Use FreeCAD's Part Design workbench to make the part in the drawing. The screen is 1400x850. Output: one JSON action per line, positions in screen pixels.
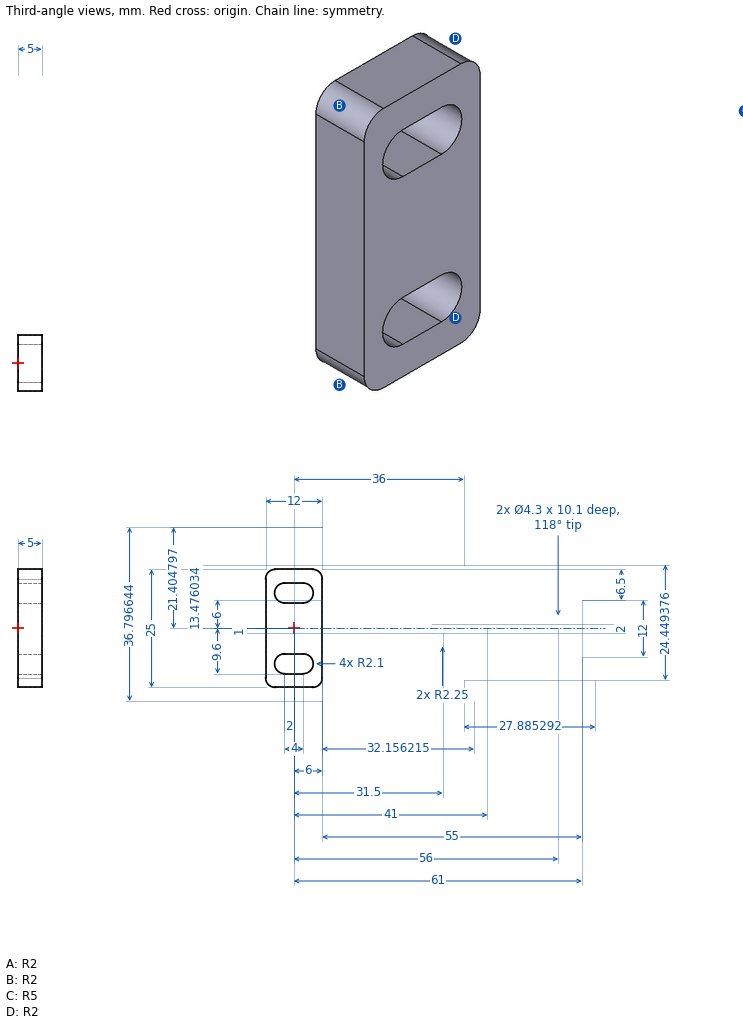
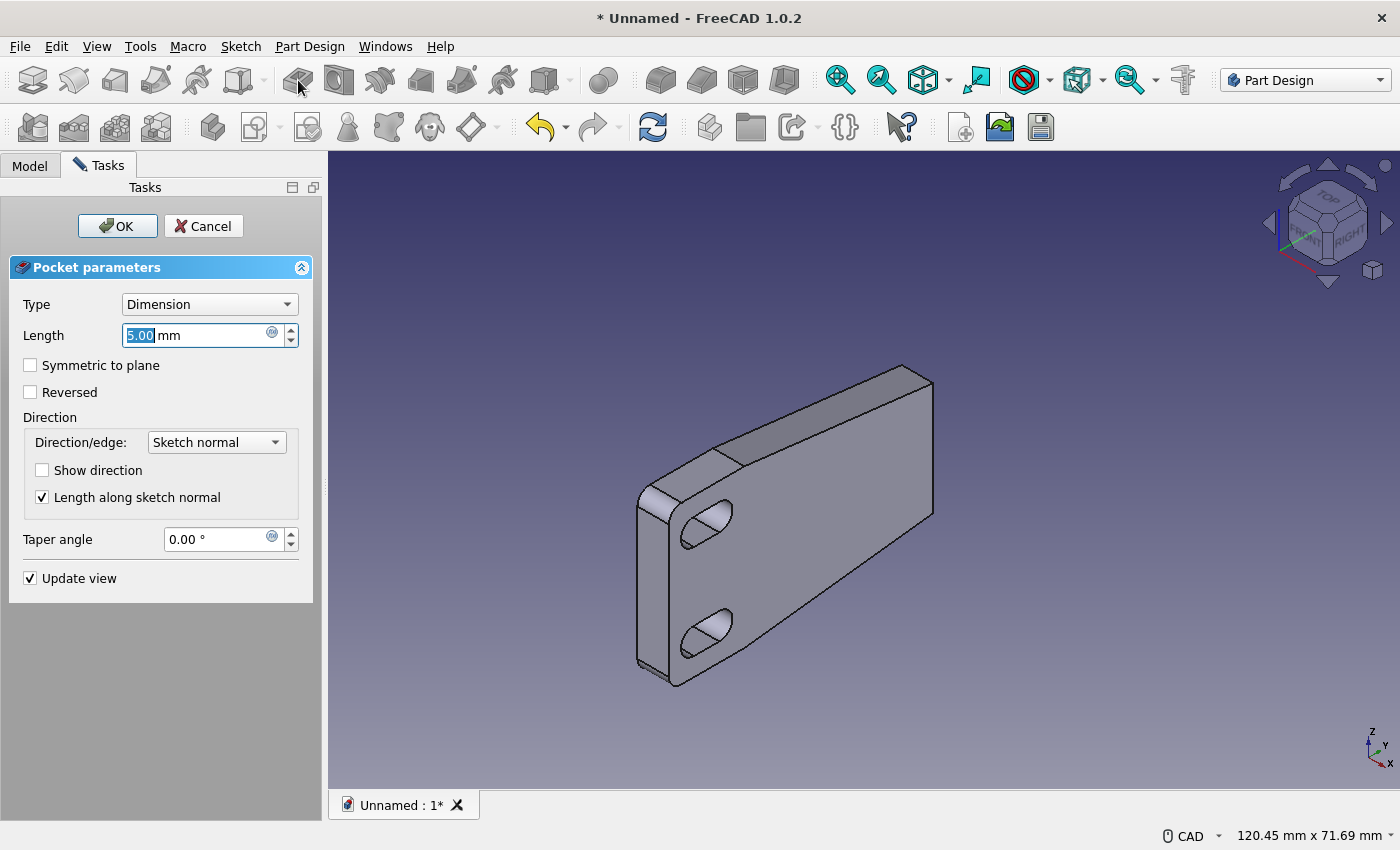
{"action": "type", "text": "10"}
{"action": "key", "text": "Tab"}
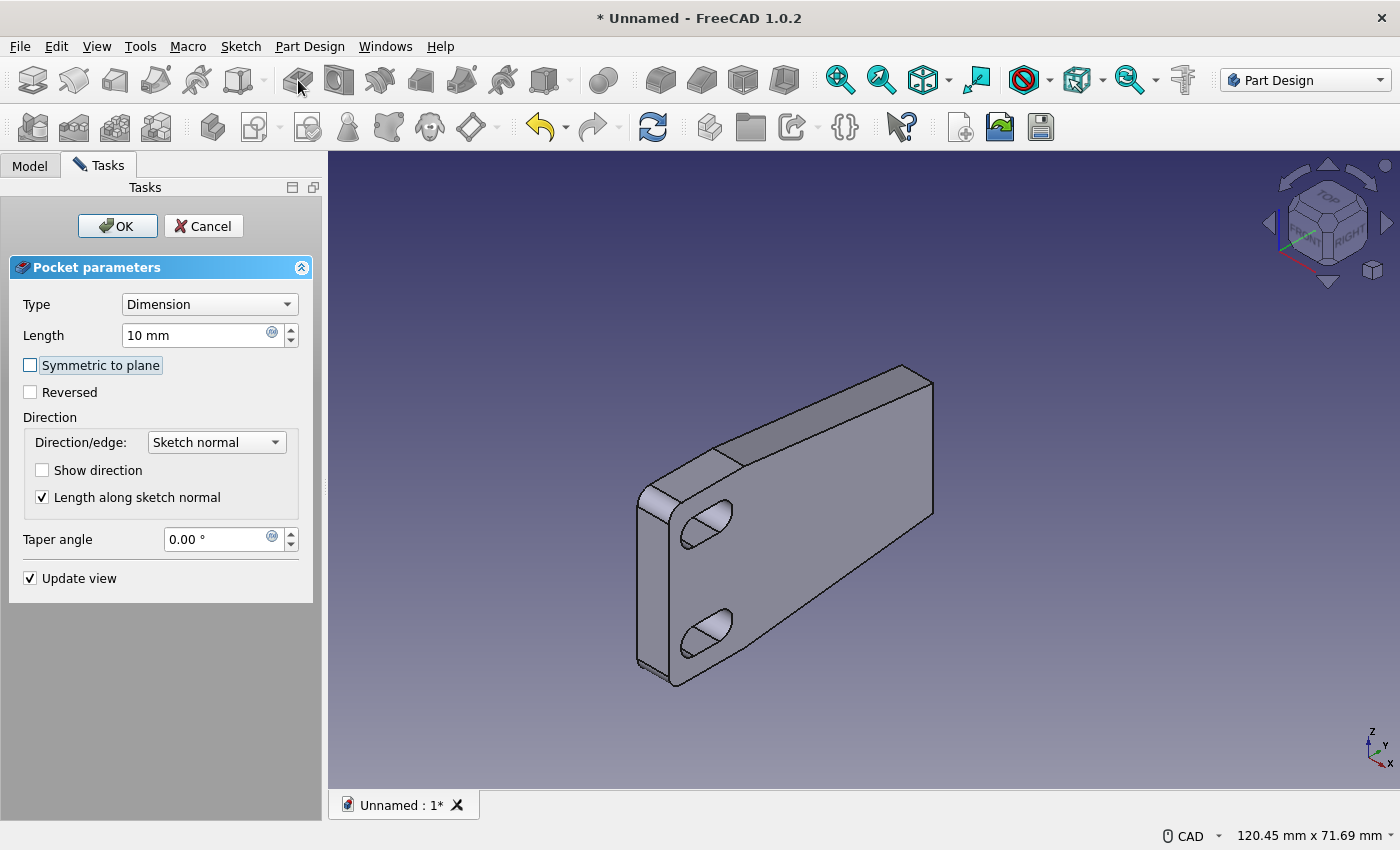
{"action": "left_click", "coordinate": [118, 226]}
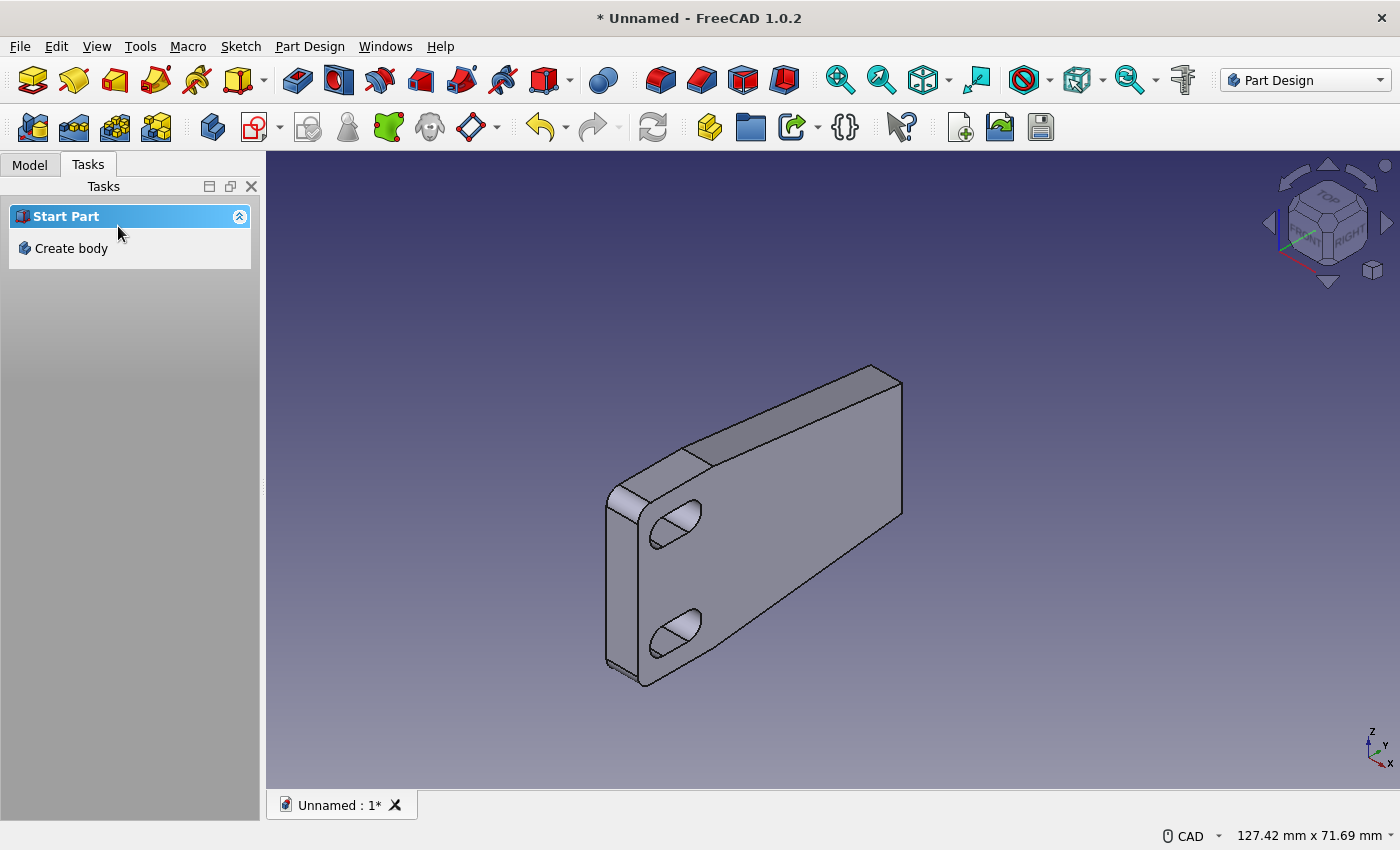
{"action": "left_click", "coordinate": [254, 128]}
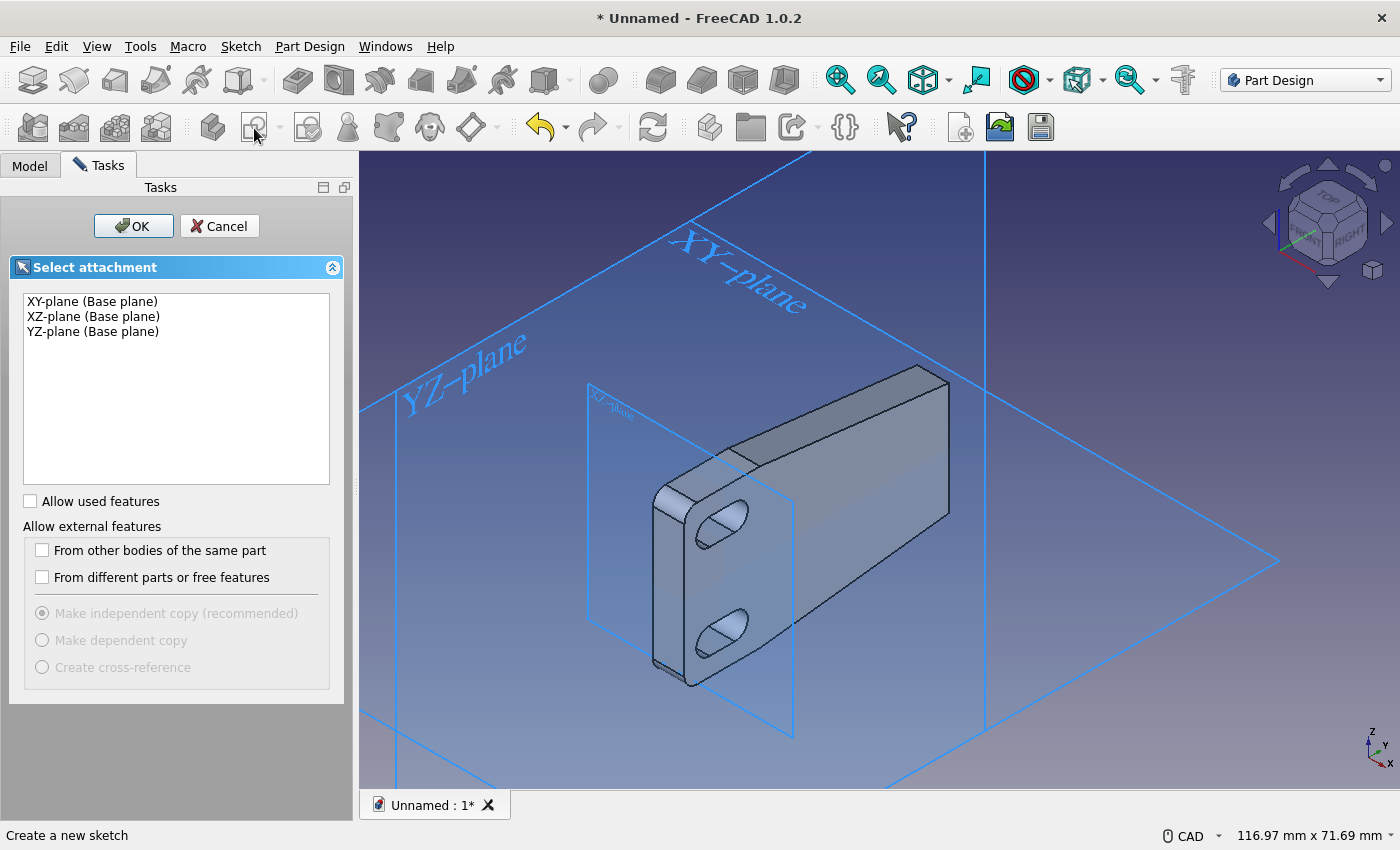
{"action": "left_click", "coordinate": [84, 332]}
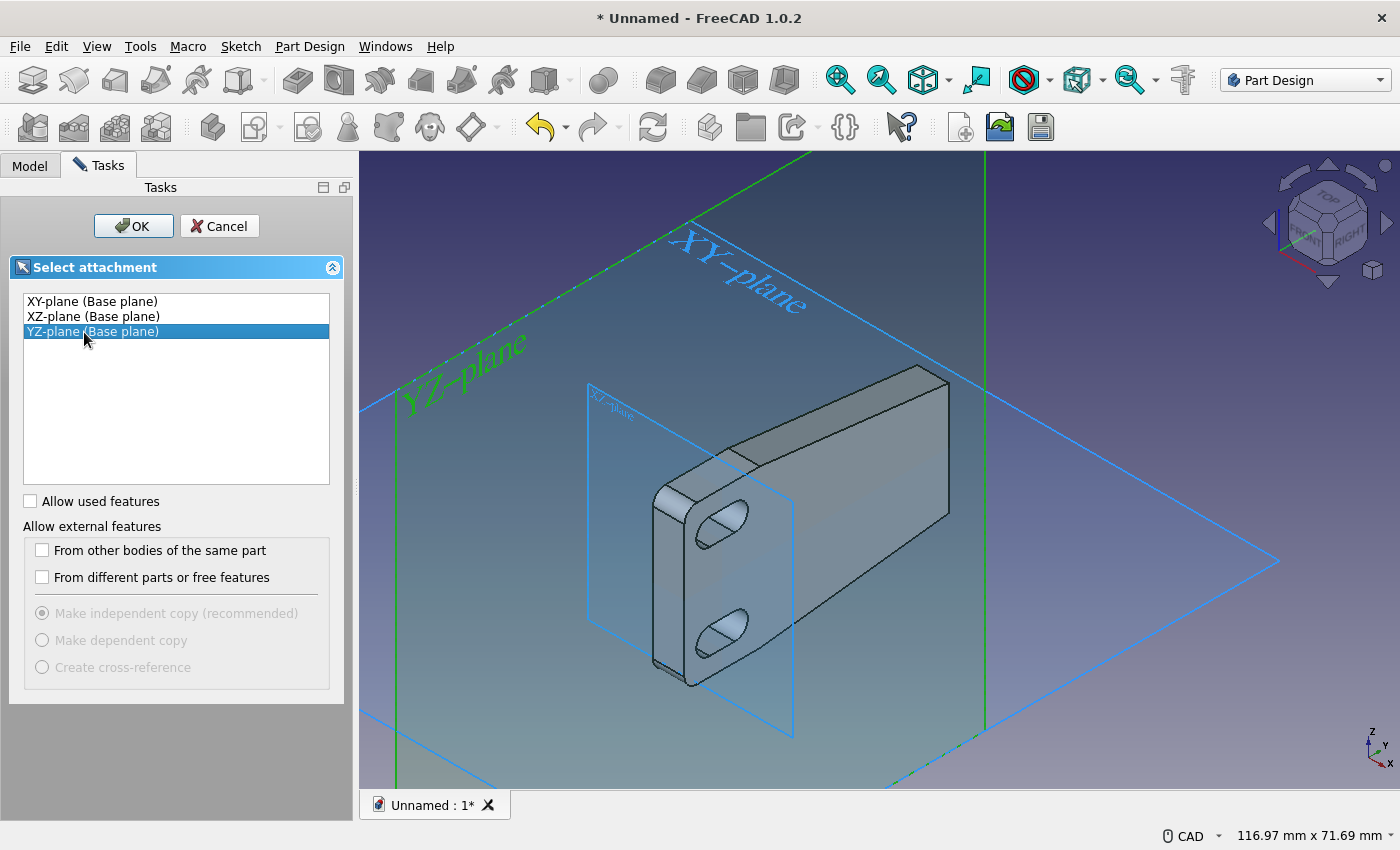
{"action": "left_click", "coordinate": [134, 226]}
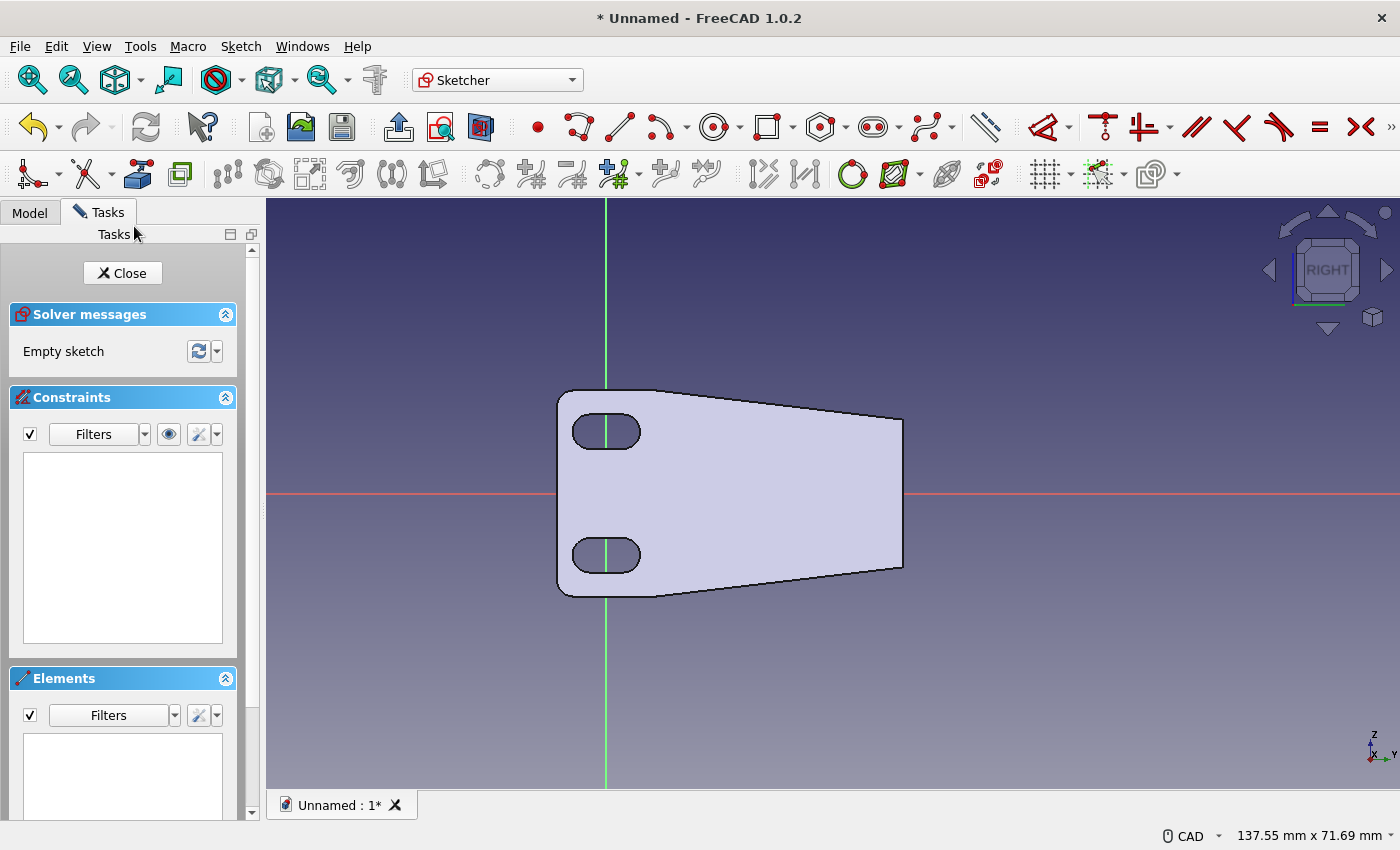
{"action": "left_click", "coordinate": [481, 128]}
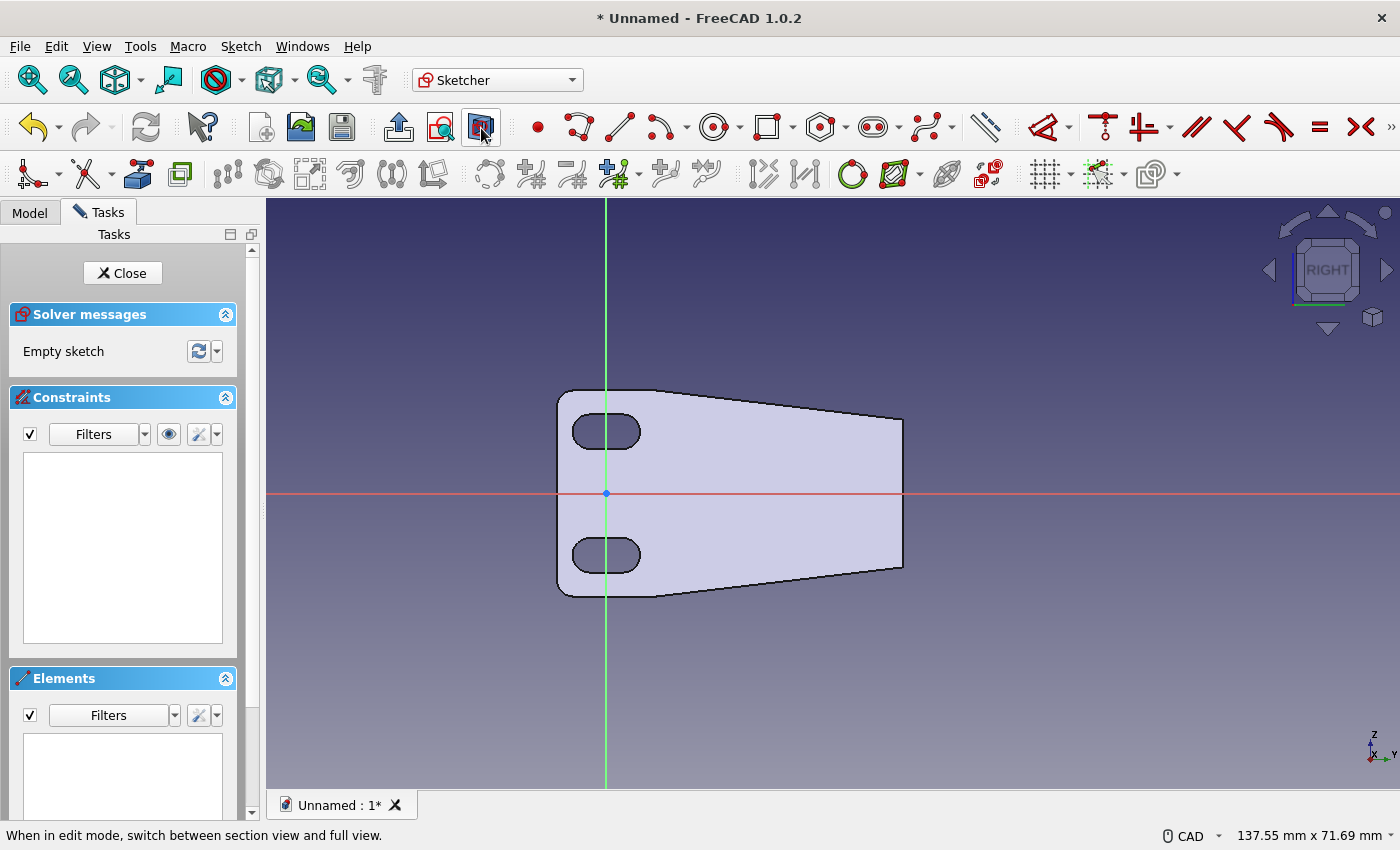
{"action": "scroll", "coordinate": [882, 493], "scroll_direction": "up", "scroll_amount": 10}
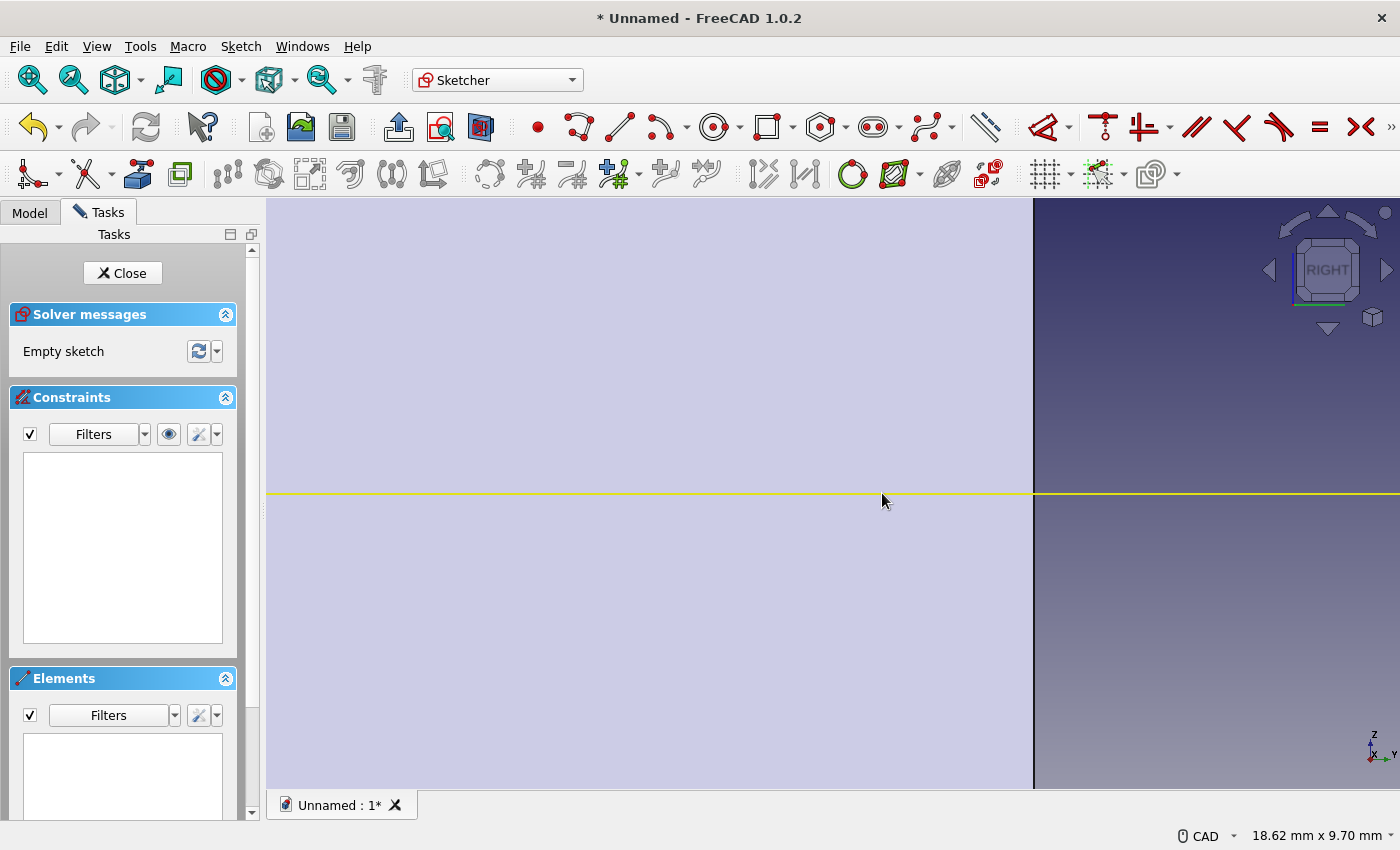
{"action": "key", "text": "g s"}